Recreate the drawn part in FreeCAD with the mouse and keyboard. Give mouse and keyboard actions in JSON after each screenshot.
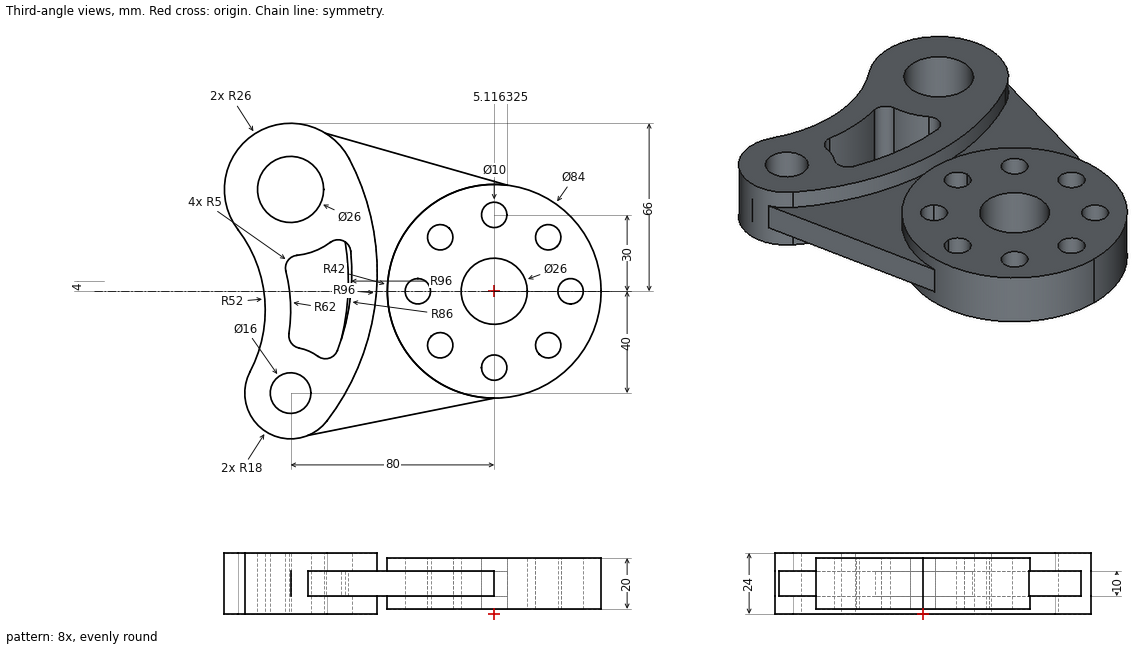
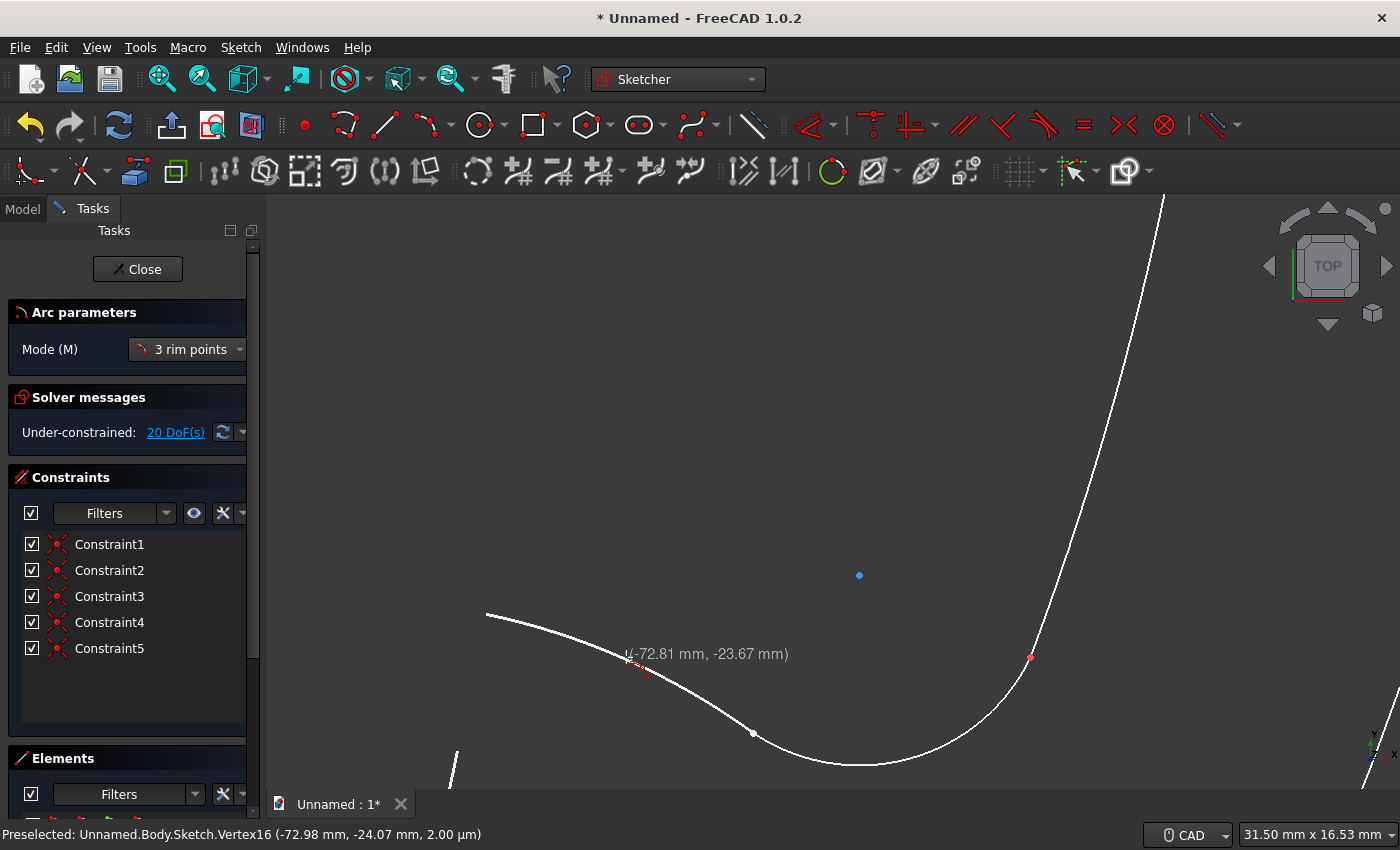
{"action": "left_click", "coordinate": [626, 653]}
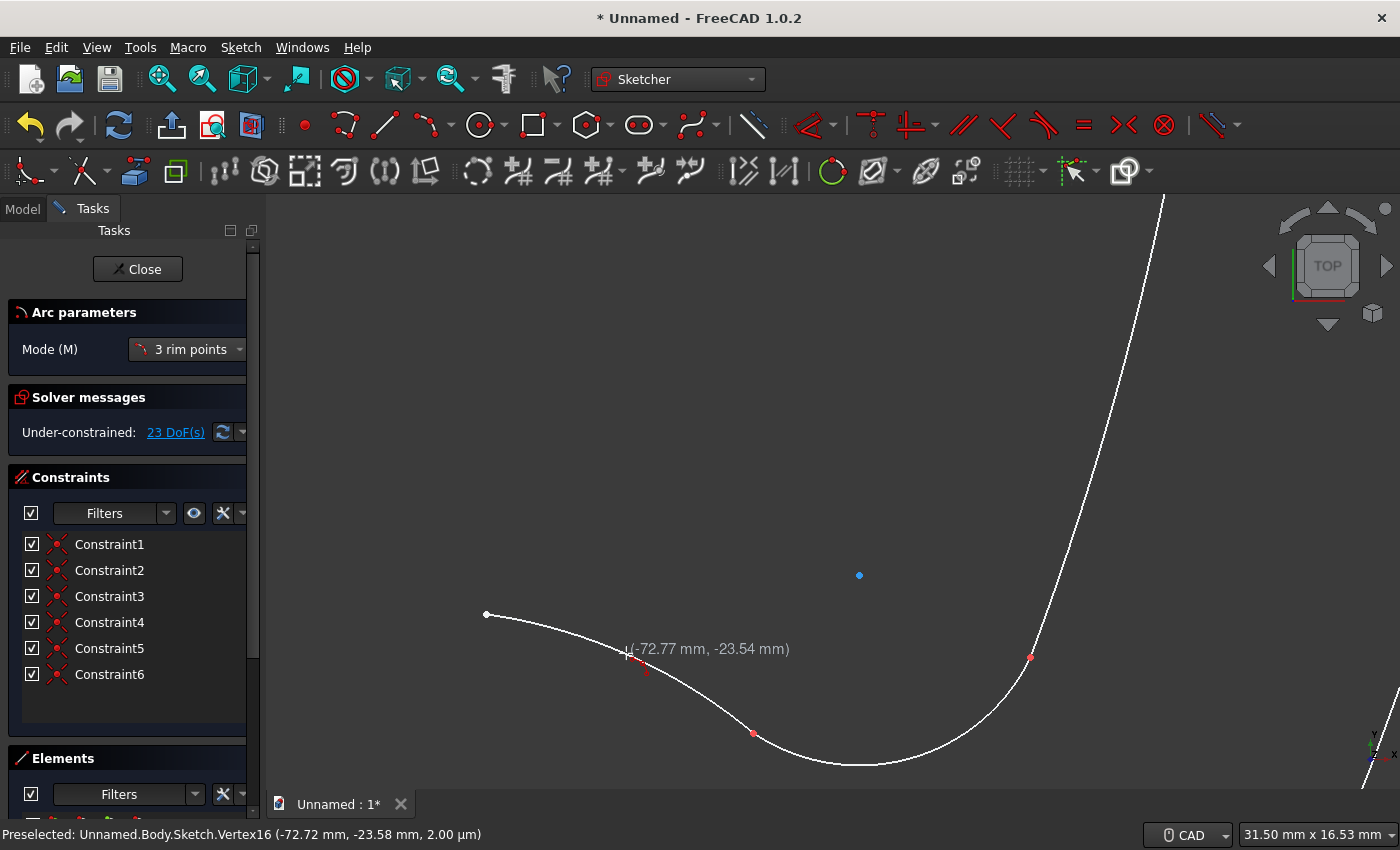
{"action": "scroll", "coordinate": [698, 572], "scroll_direction": "down", "scroll_amount": 12}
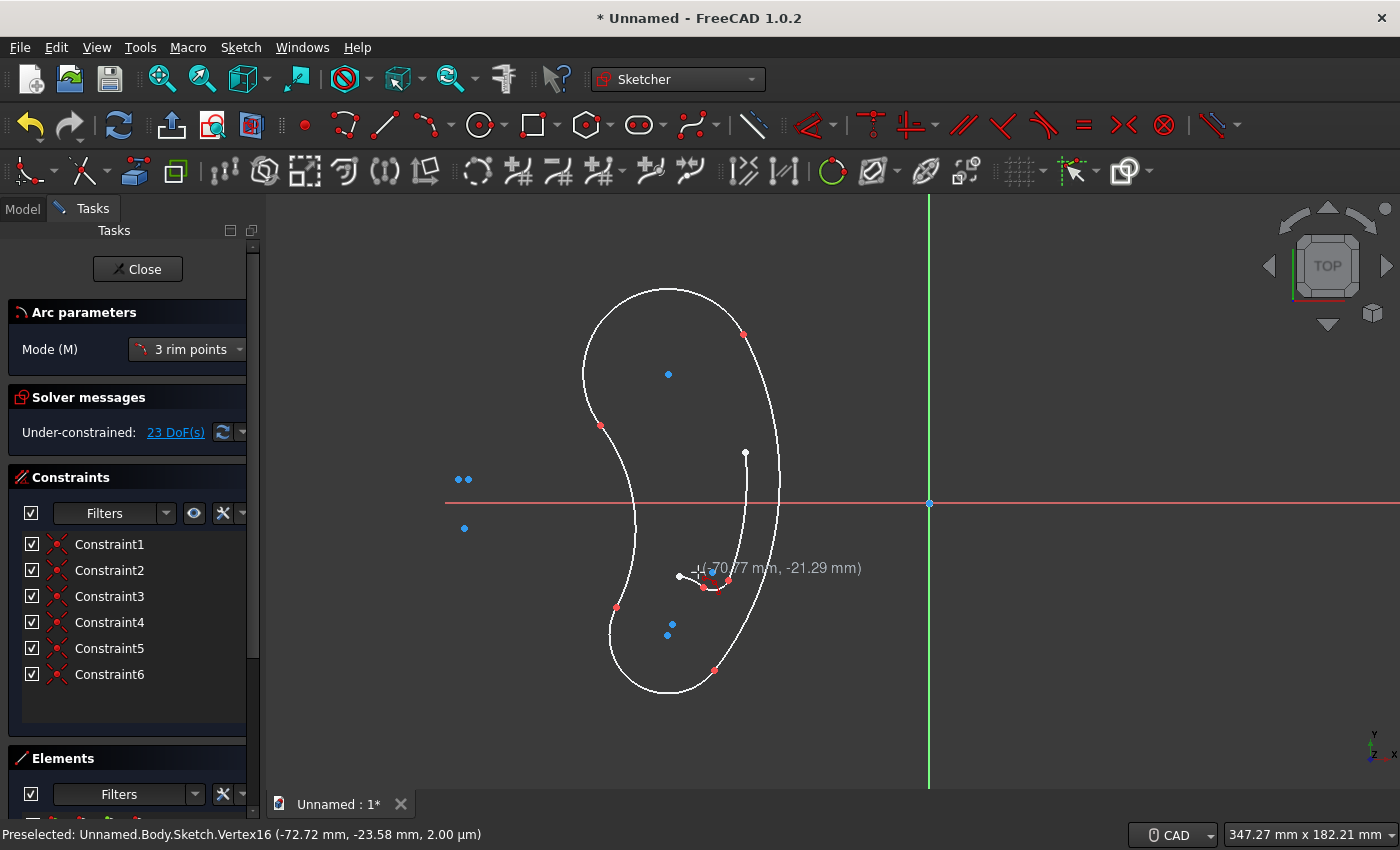
{"action": "left_click", "coordinate": [679, 576]}
{"action": "left_click", "coordinate": [666, 558]}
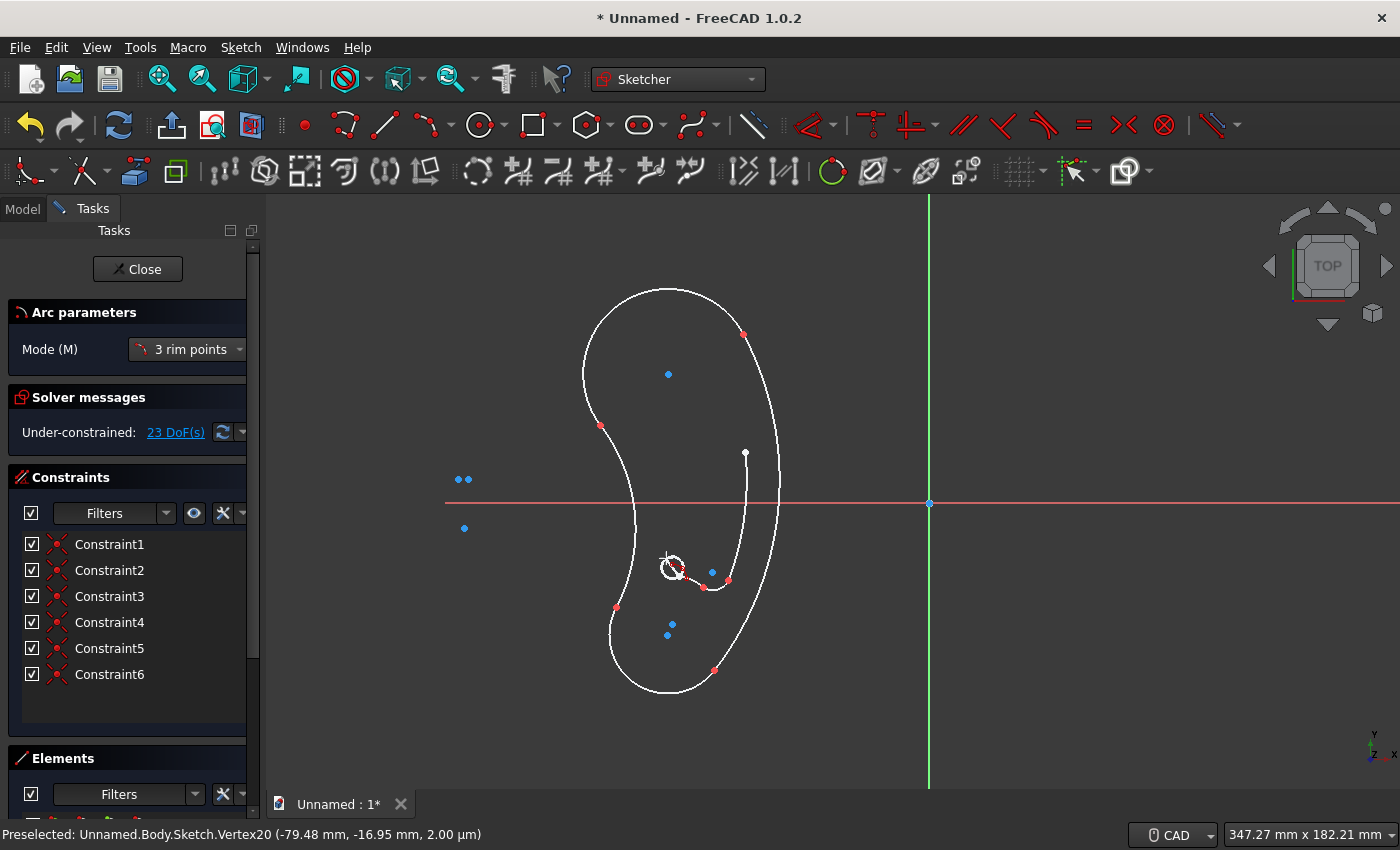
{"action": "scroll", "coordinate": [669, 569], "scroll_direction": "up", "scroll_amount": 7}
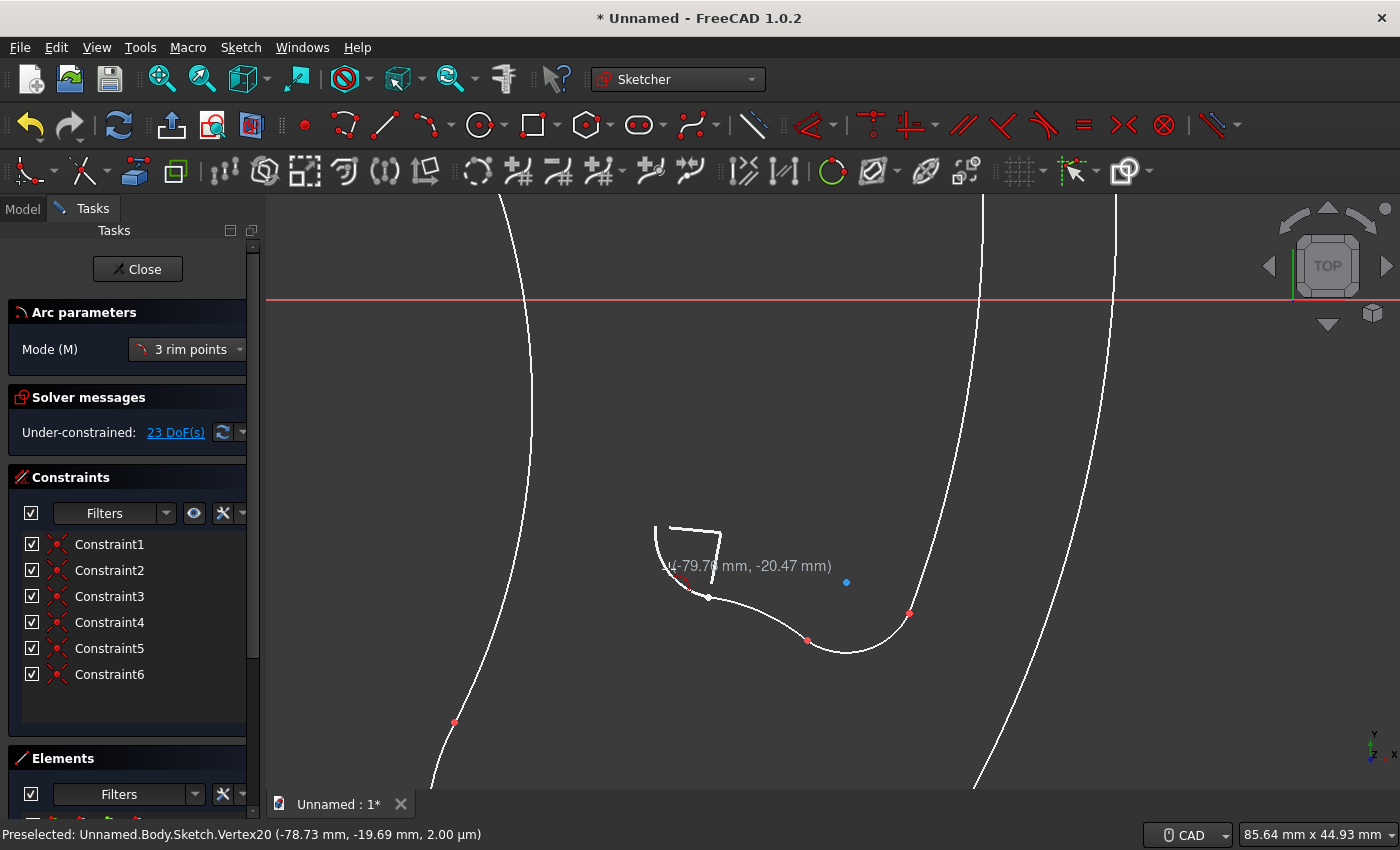
{"action": "left_click", "coordinate": [668, 569]}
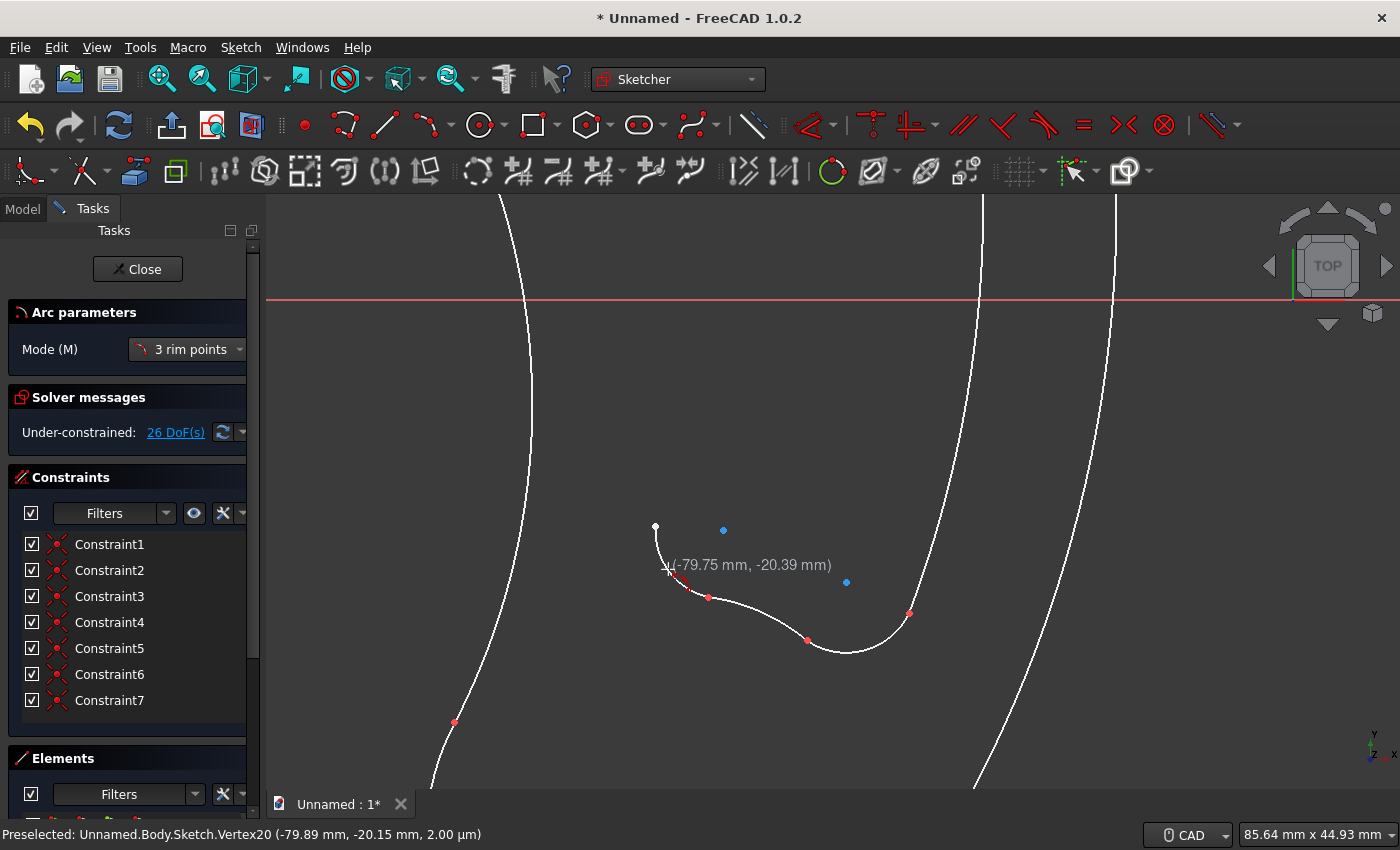
{"action": "scroll", "coordinate": [669, 569], "scroll_direction": "down", "scroll_amount": 7}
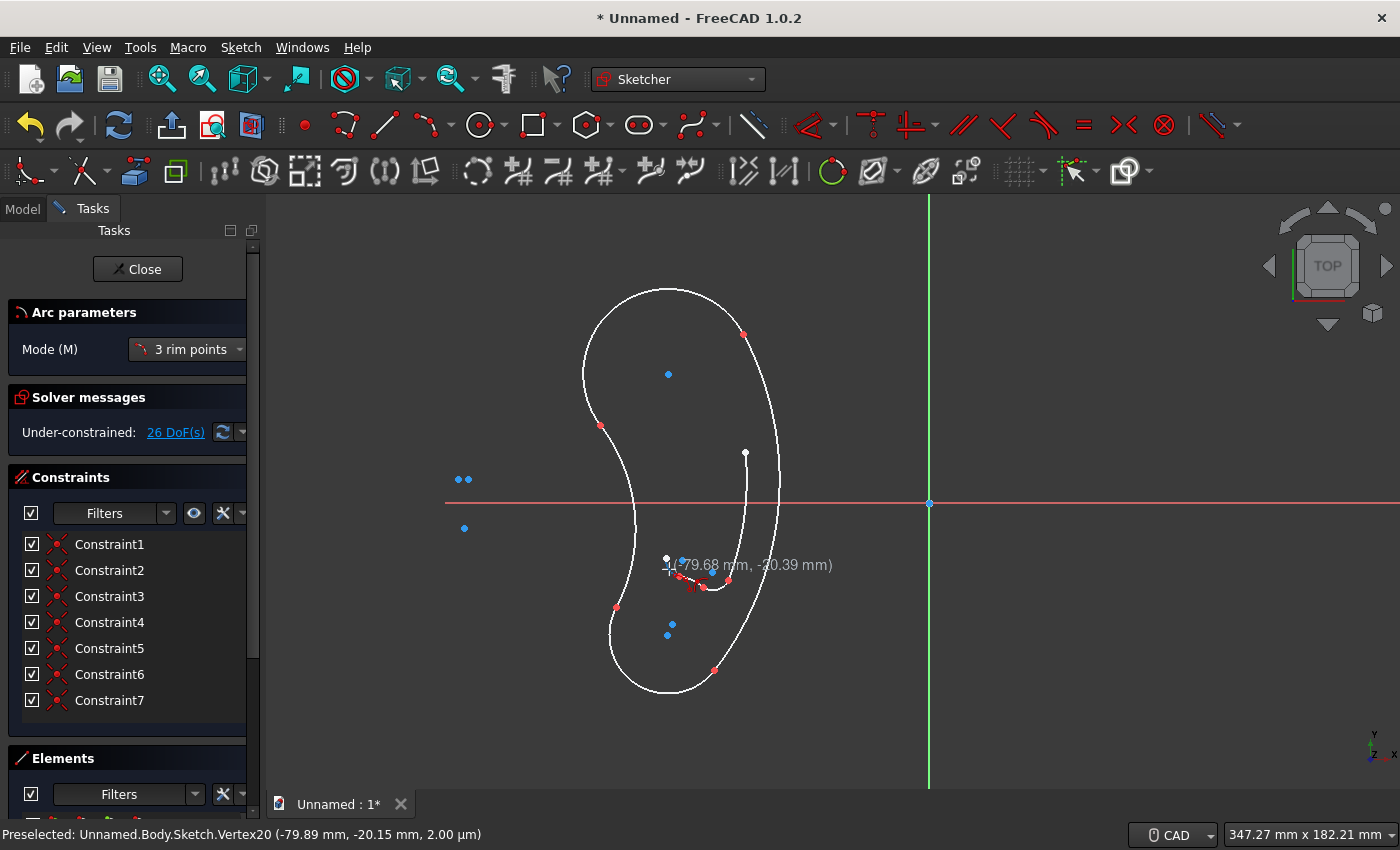
{"action": "left_click", "coordinate": [666, 559]}
{"action": "left_click", "coordinate": [662, 477]}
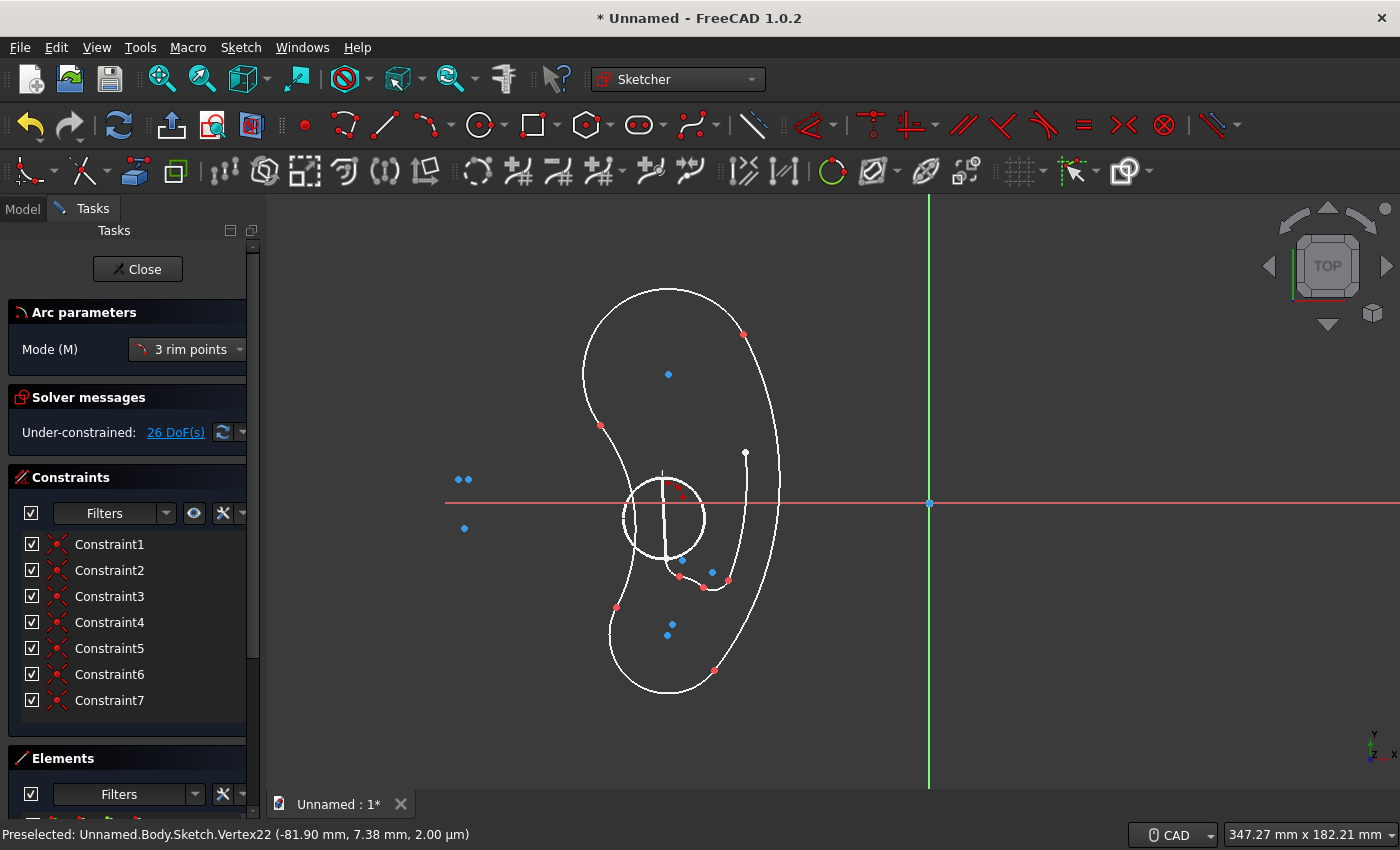
{"action": "scroll", "coordinate": [668, 517], "scroll_direction": "up", "scroll_amount": 7}